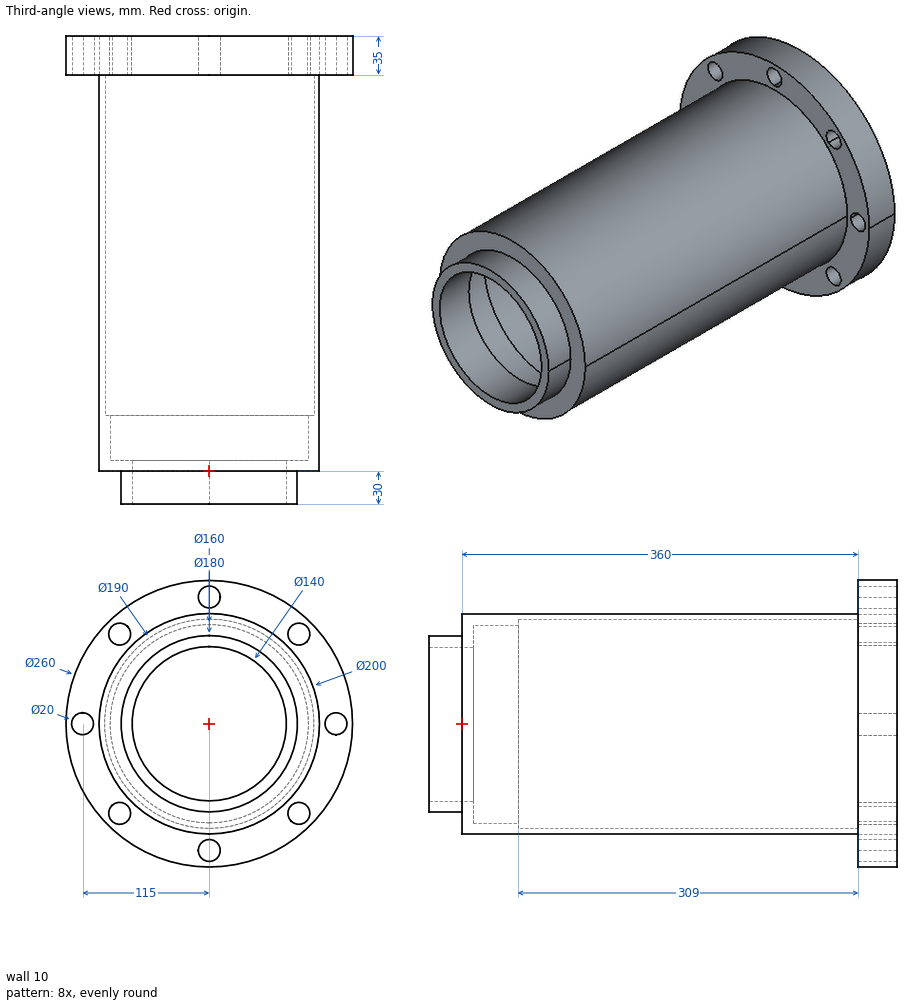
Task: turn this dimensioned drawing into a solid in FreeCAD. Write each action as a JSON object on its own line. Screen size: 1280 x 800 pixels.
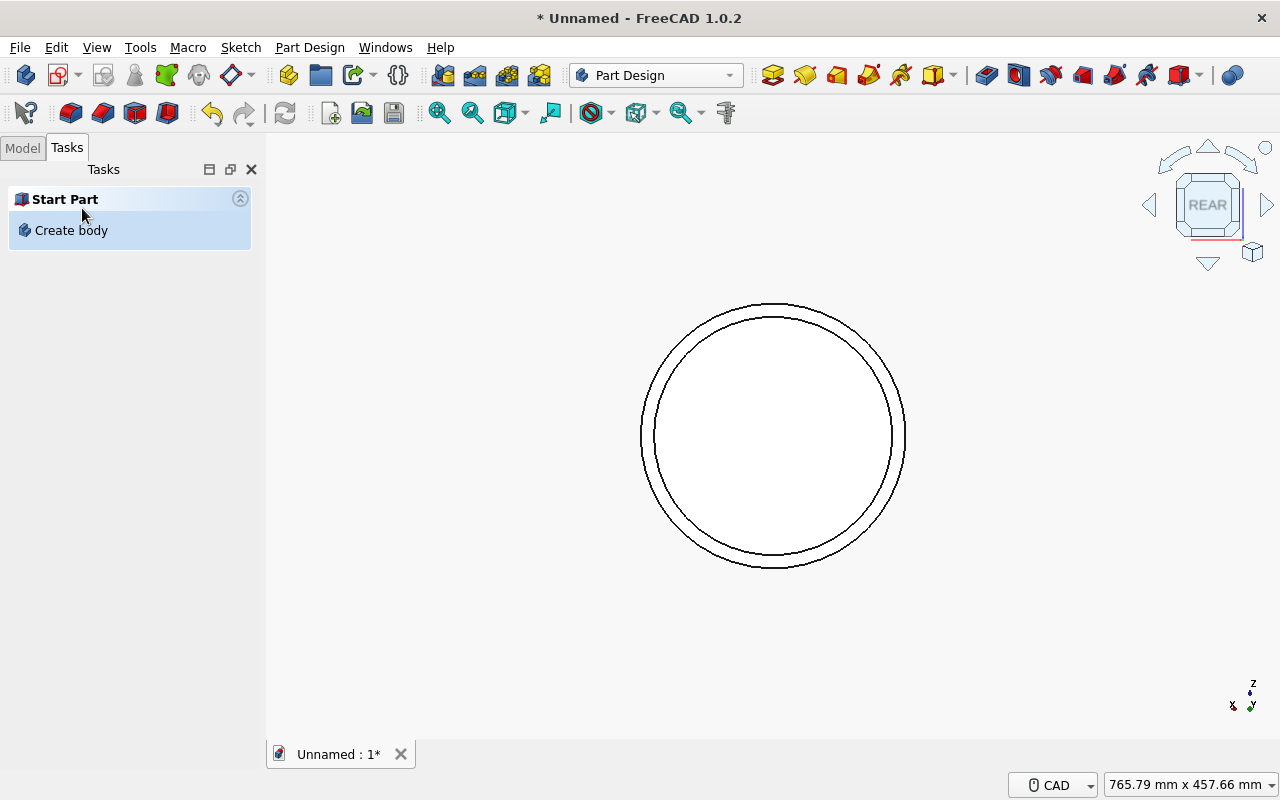
{"action": "key", "text": "v f"}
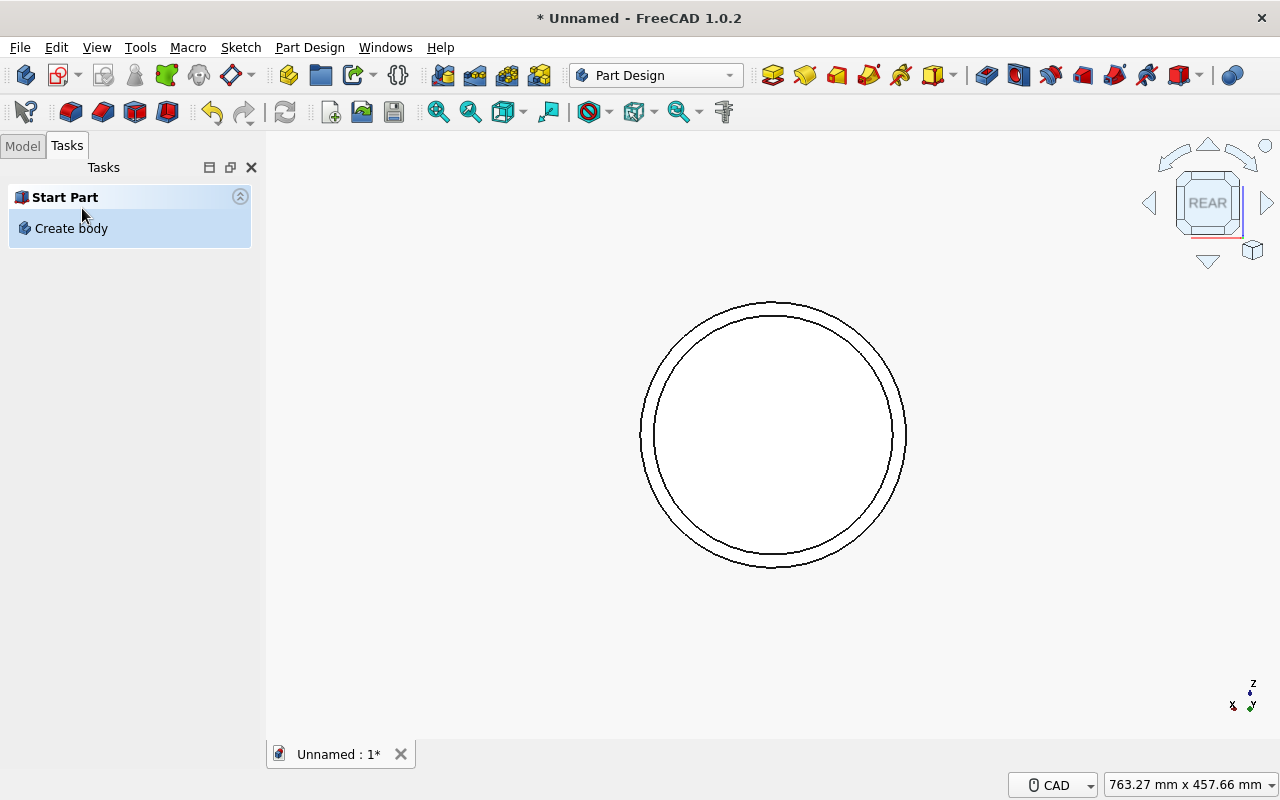
{"action": "left_click", "coordinate": [773, 434]}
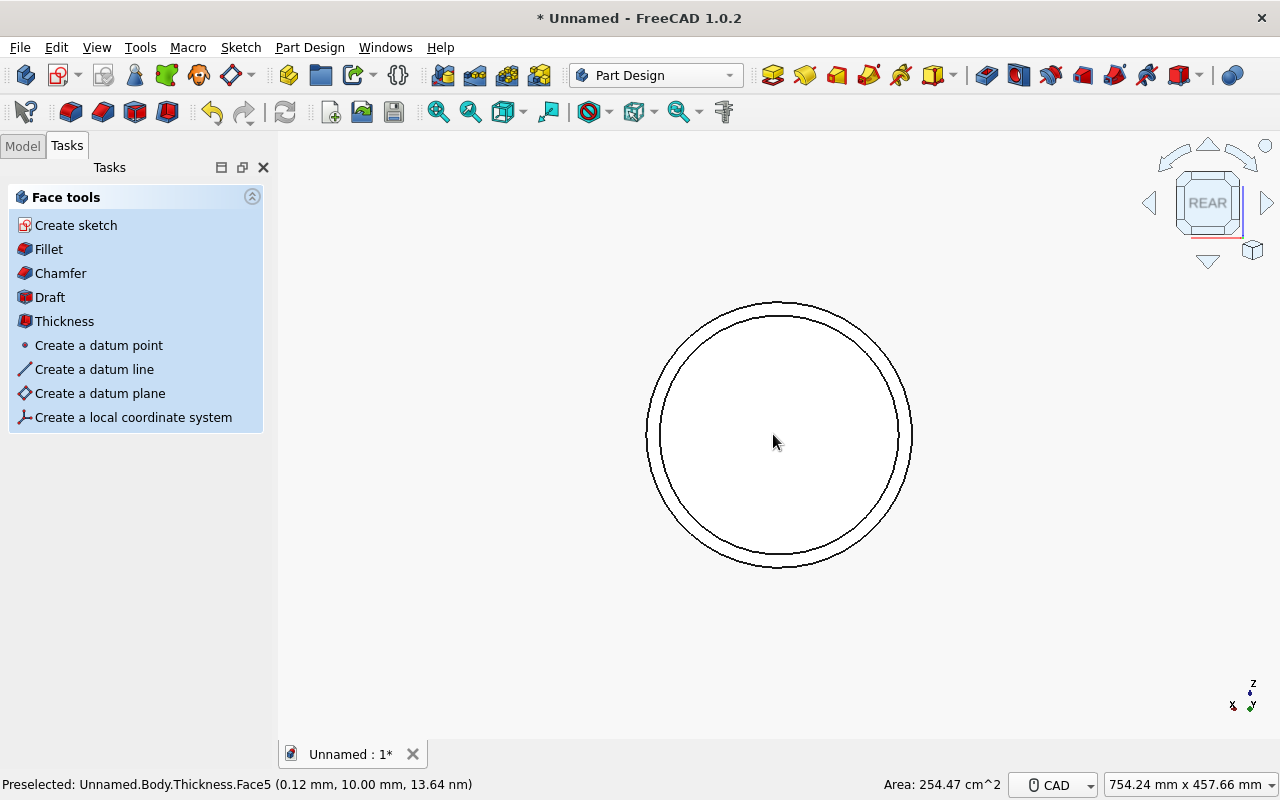
{"action": "left_click", "coordinate": [58, 76]}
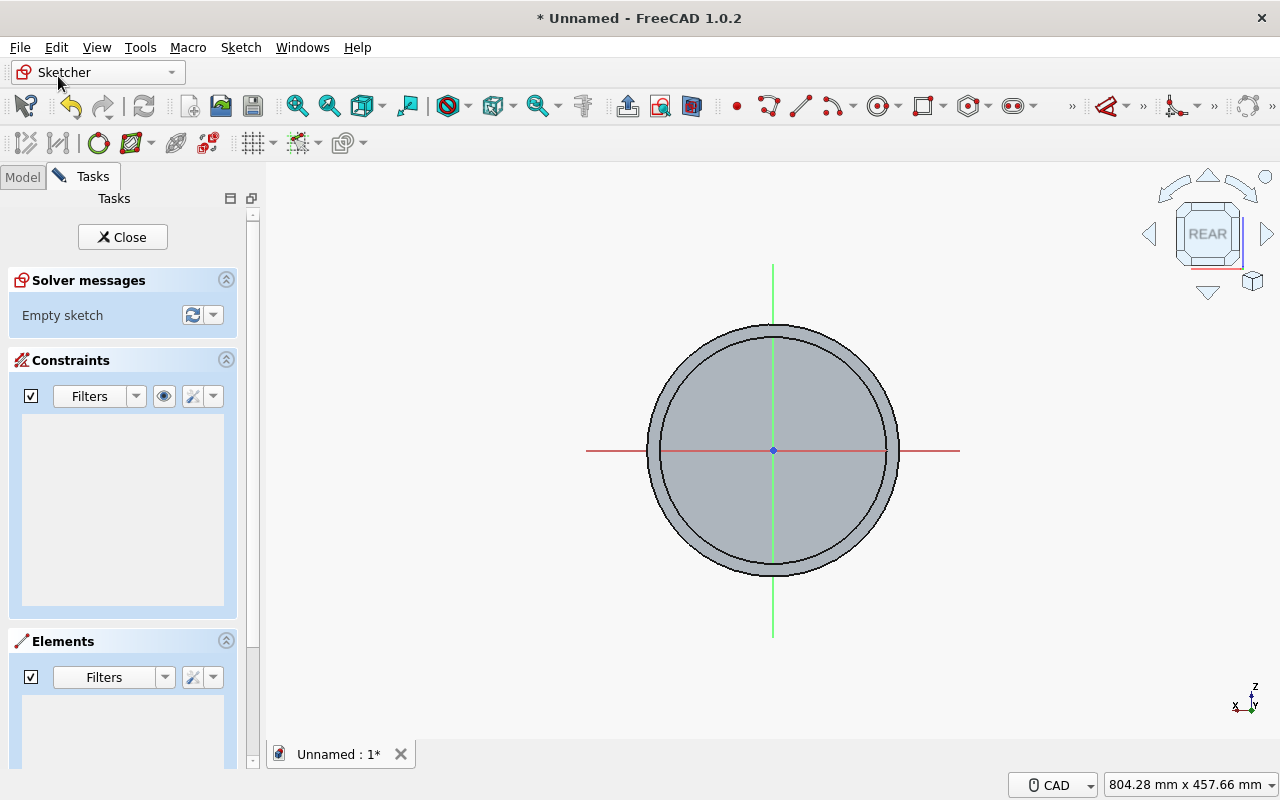
{"action": "left_click", "coordinate": [692, 106]}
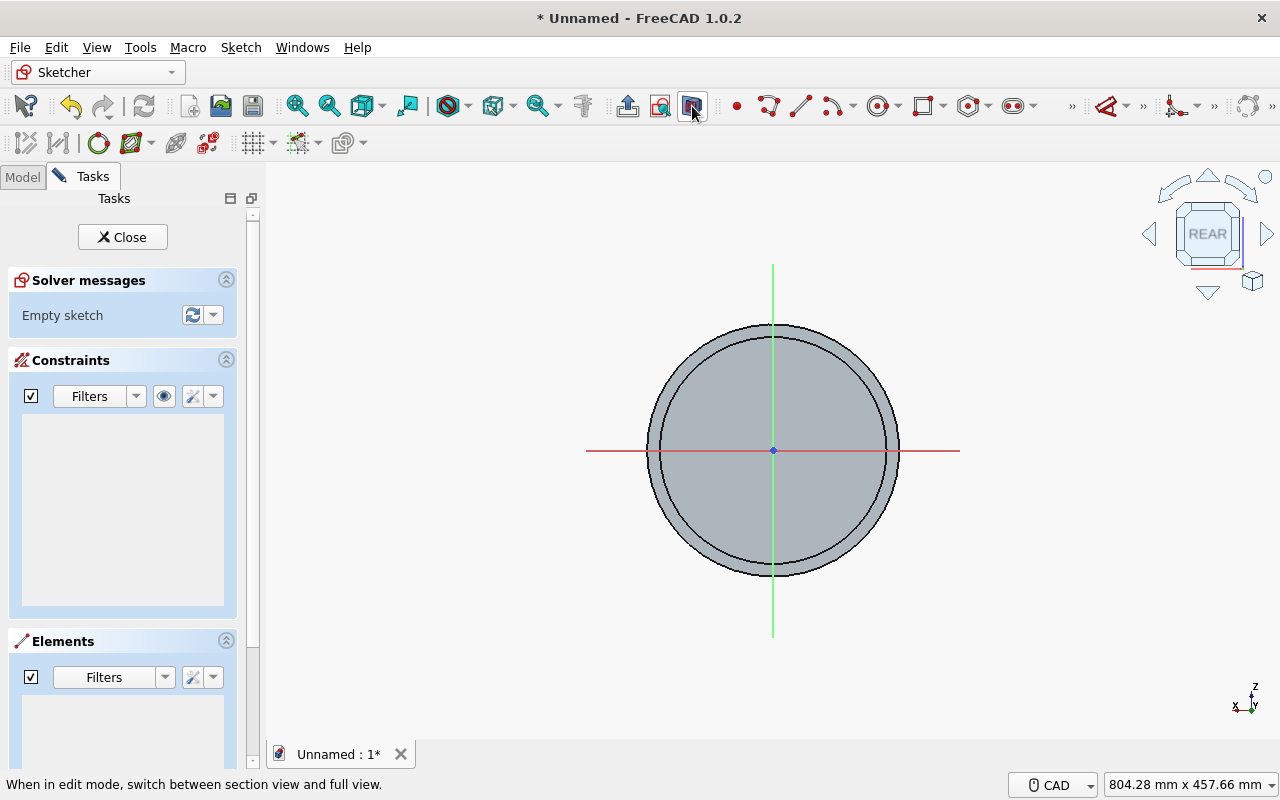
{"action": "scroll", "coordinate": [829, 450], "scroll_direction": "up", "scroll_amount": 4}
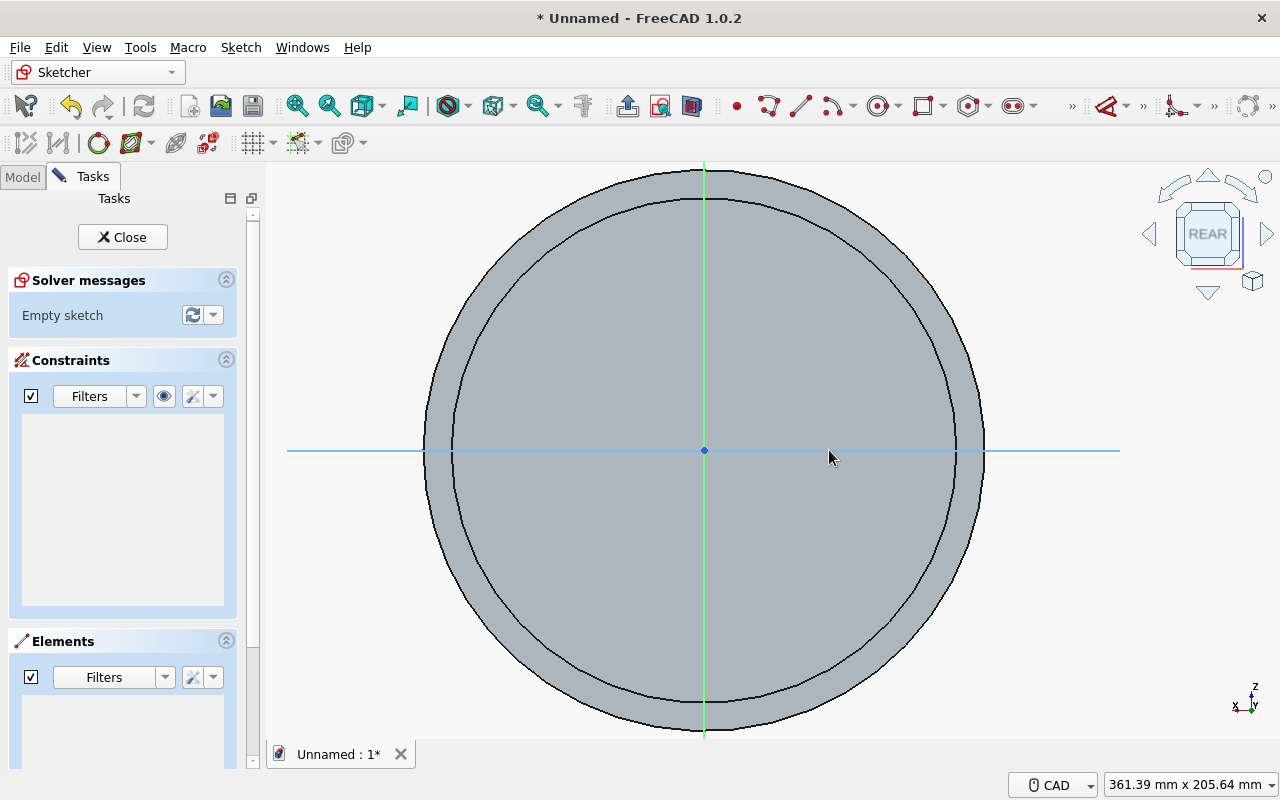
{"action": "key", "text": "g c"}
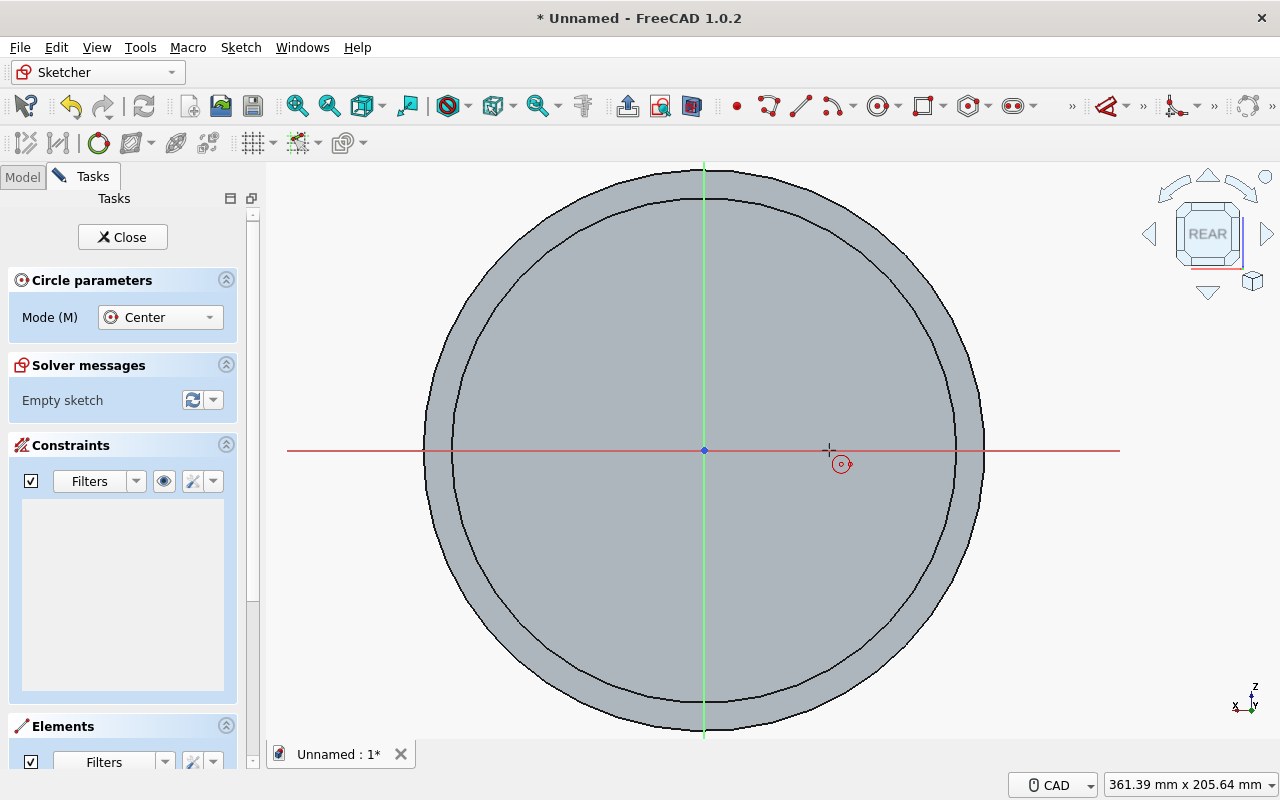
{"action": "left_click", "coordinate": [704, 450]}
{"action": "left_click", "coordinate": [843, 312]}
{"action": "key", "text": "Escape"}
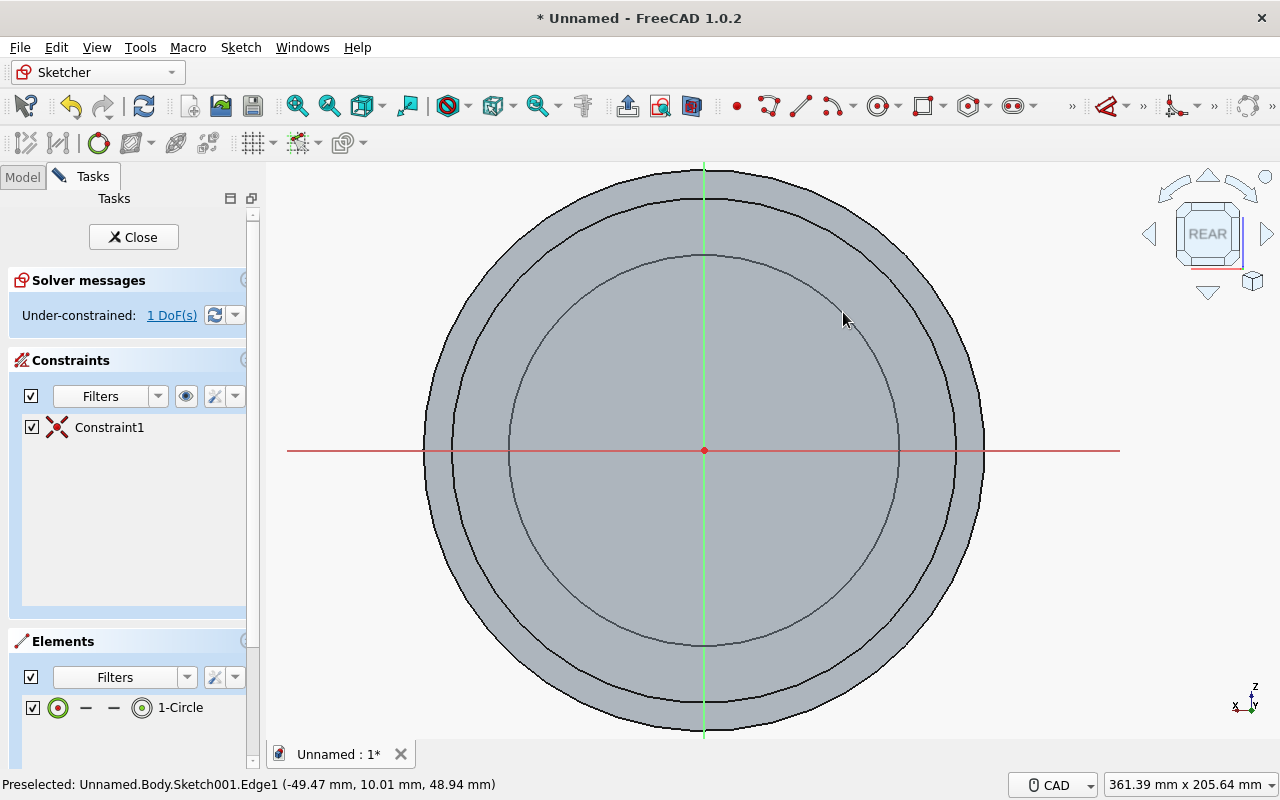
{"action": "key", "text": "d"}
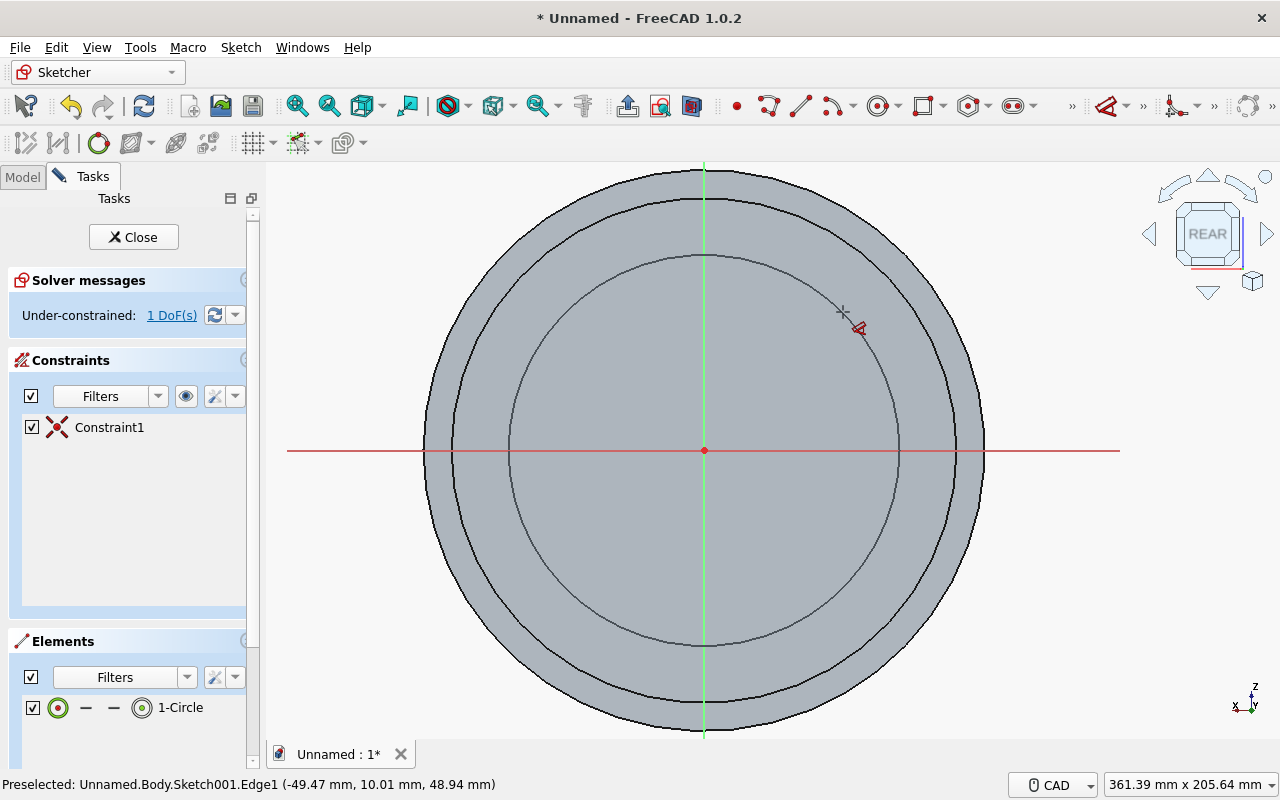
{"action": "left_click", "coordinate": [842, 312]}
{"action": "left_click", "coordinate": [865, 289]}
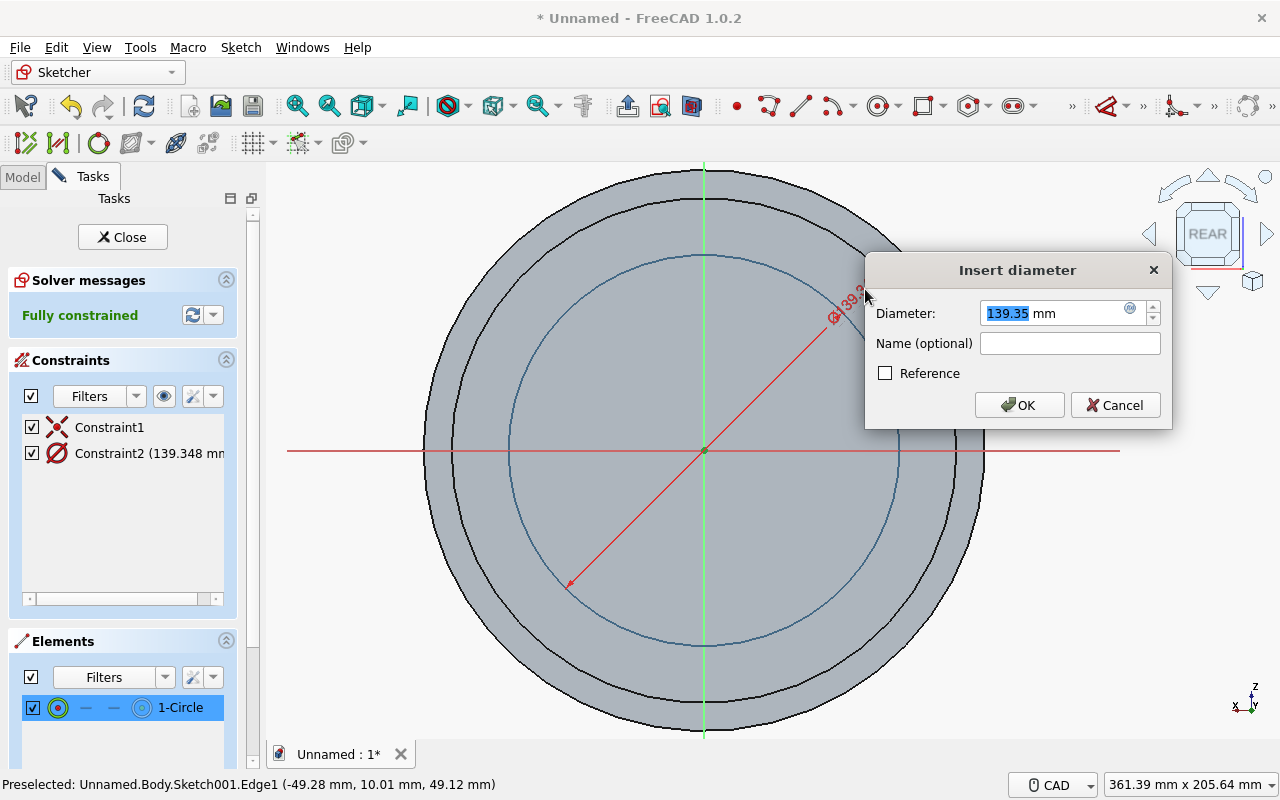
{"action": "type", "text": "140"}
{"action": "key", "text": "Return"}
{"action": "key", "text": "Escape"}